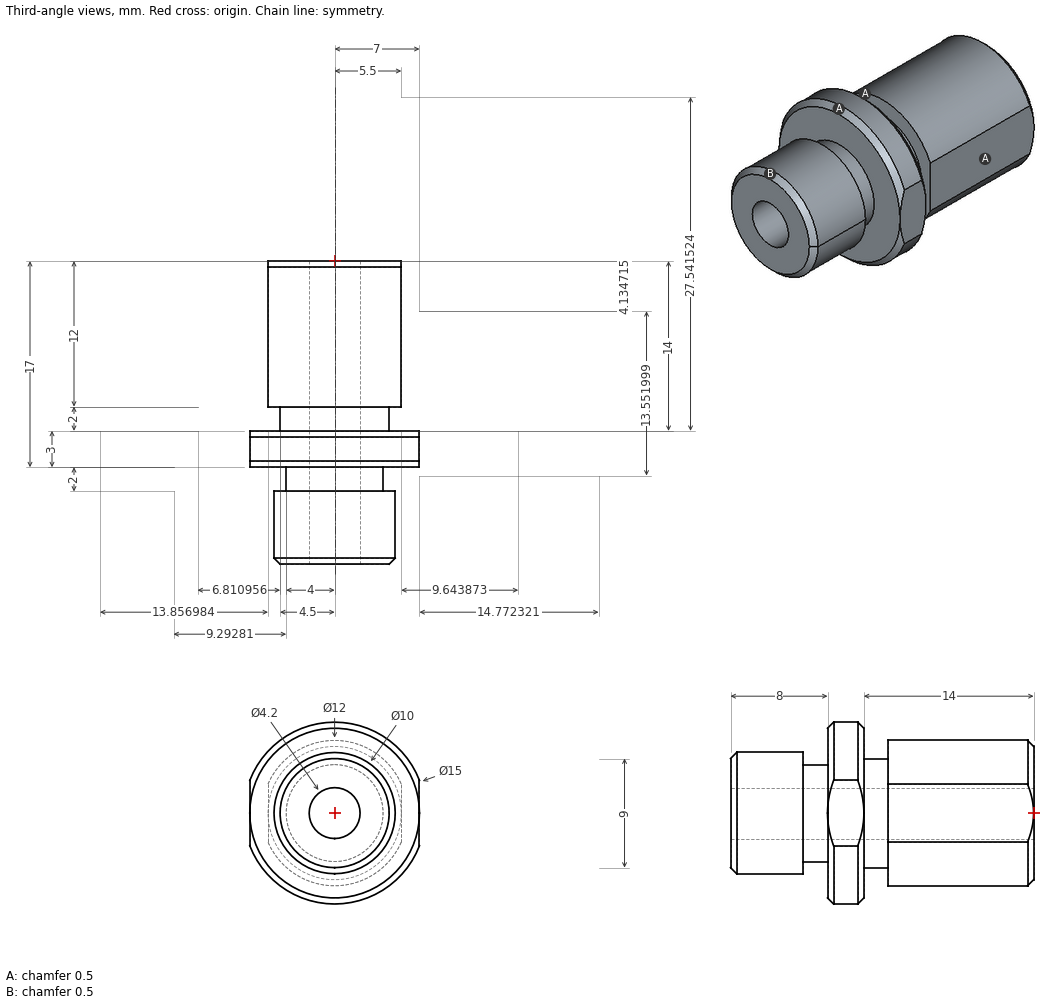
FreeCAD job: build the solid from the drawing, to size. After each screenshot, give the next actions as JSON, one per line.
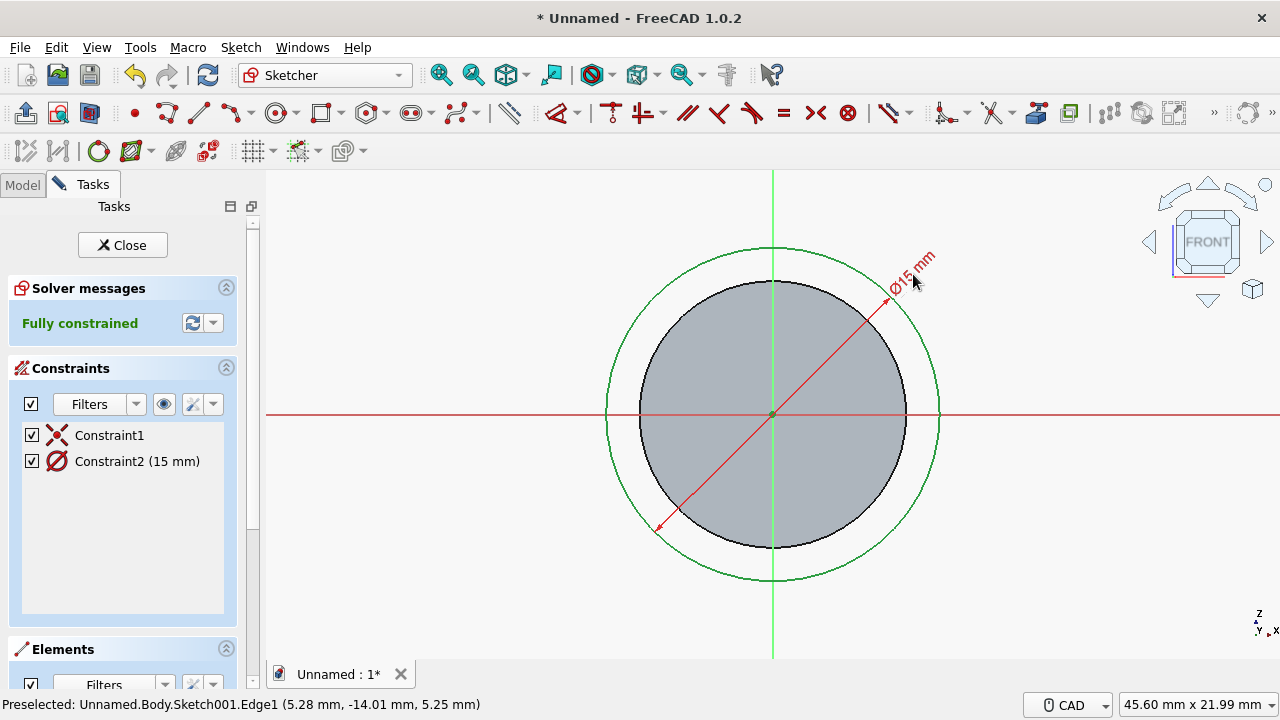
{"action": "left_click", "coordinate": [123, 245]}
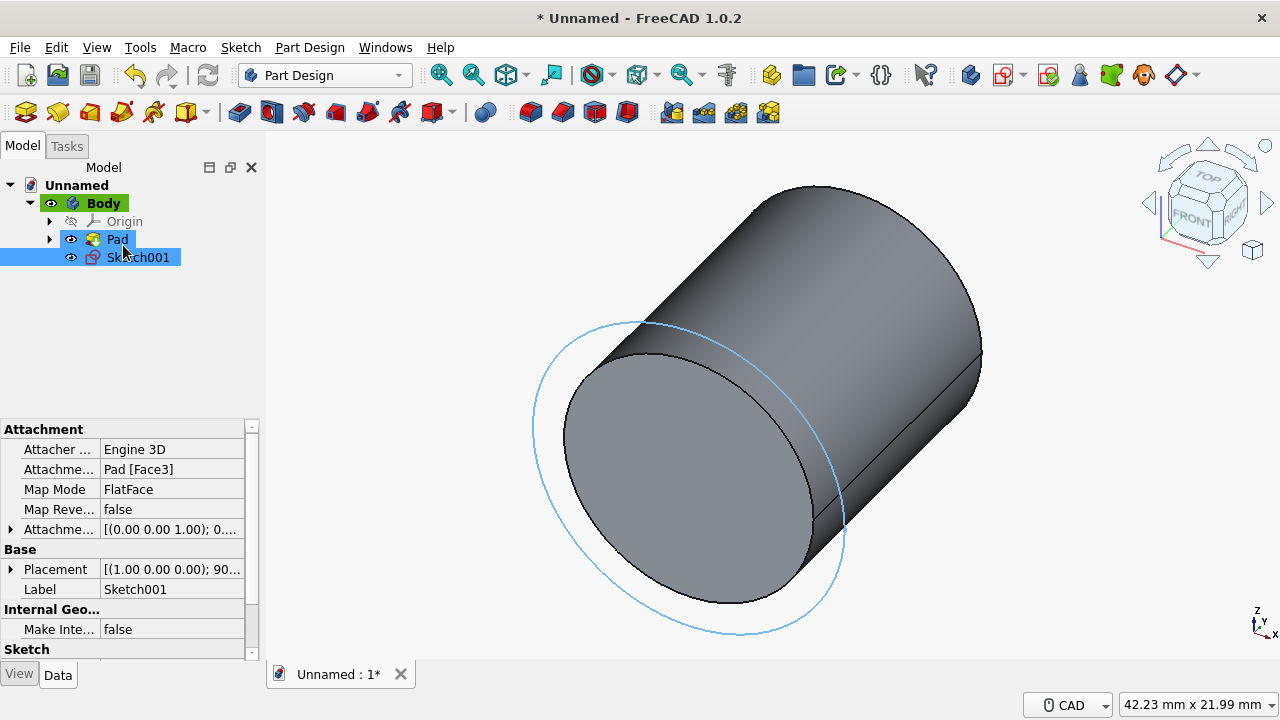
{"action": "left_click", "coordinate": [26, 112]}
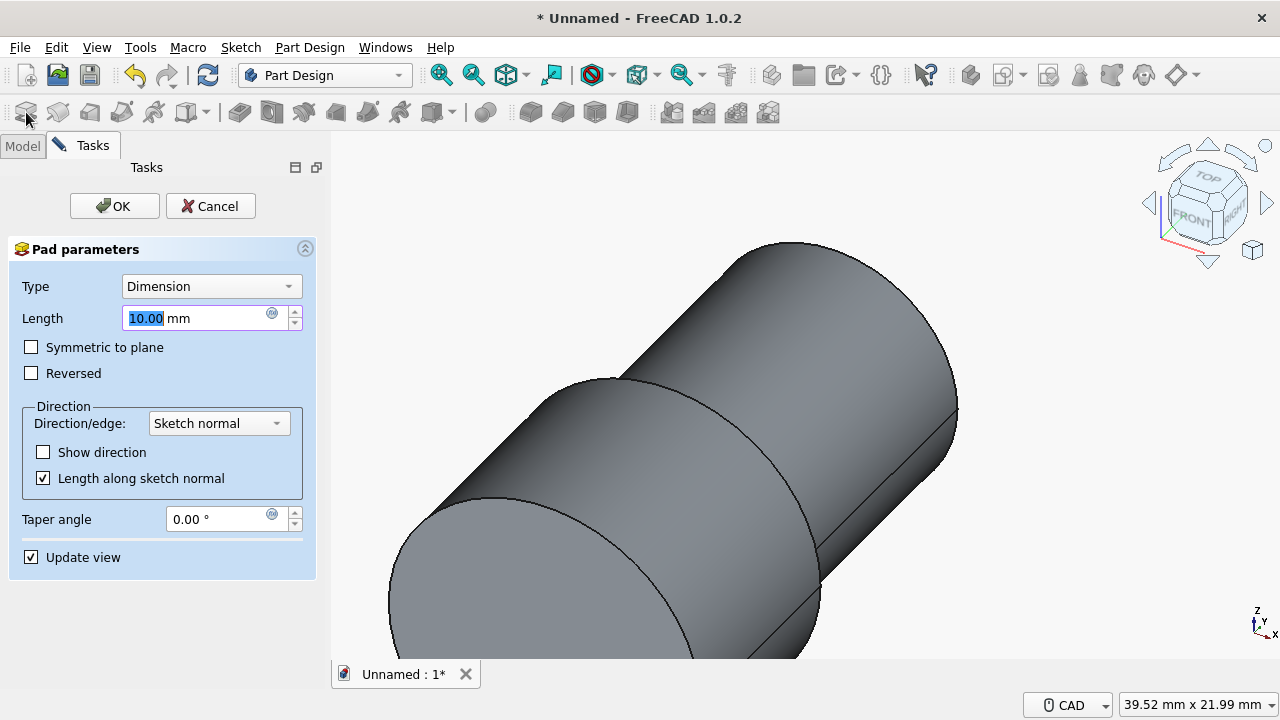
{"action": "type", "text": "3"}
{"action": "key", "text": "Tab"}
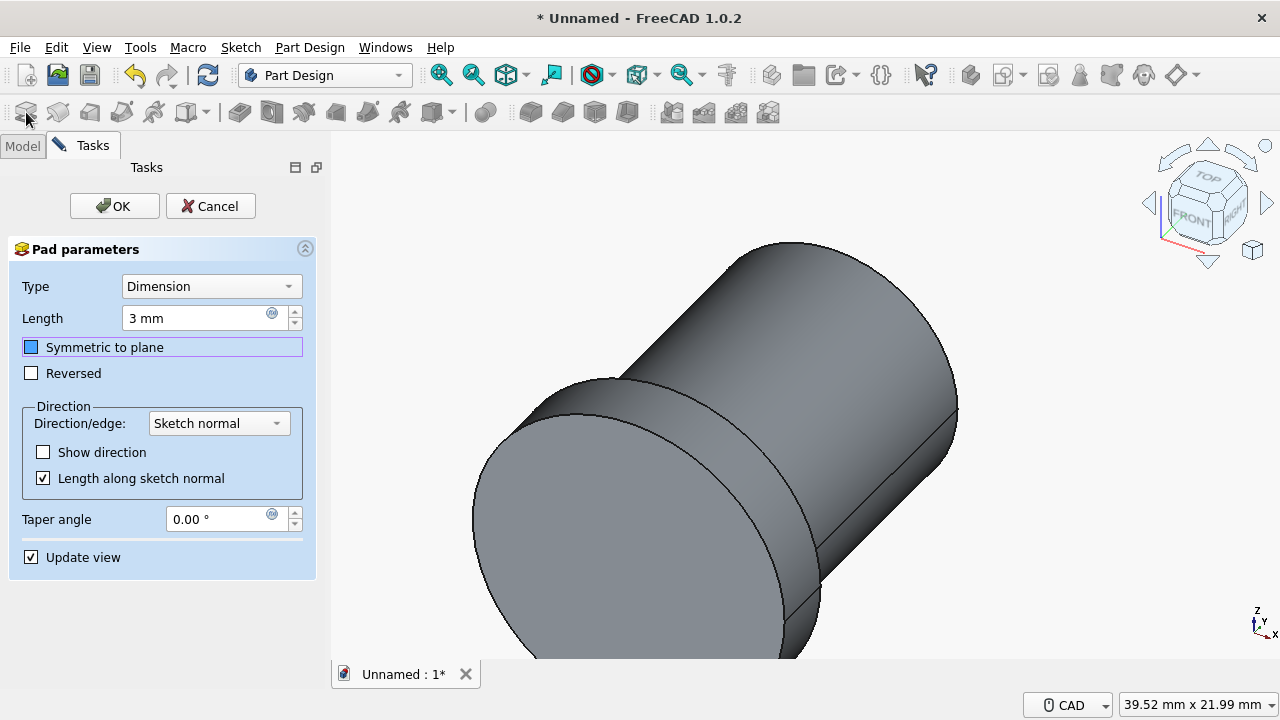
{"action": "left_click", "coordinate": [115, 206]}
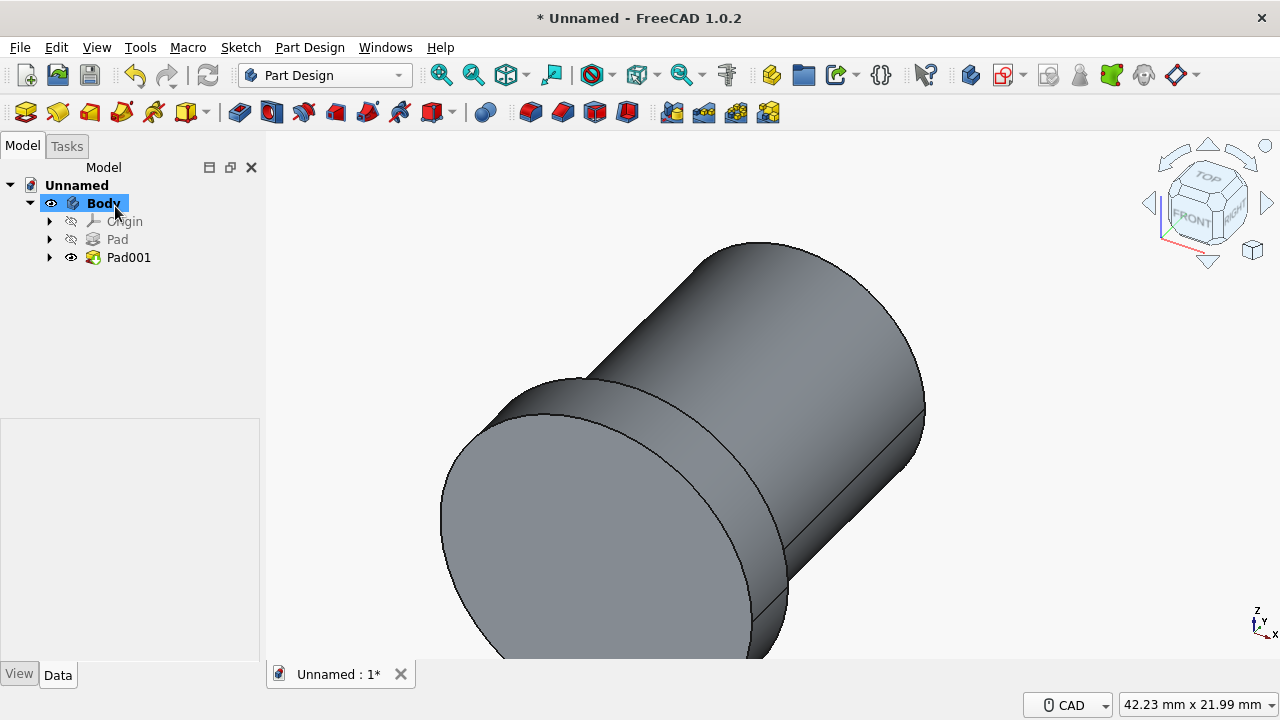
{"action": "key", "text": "v f"}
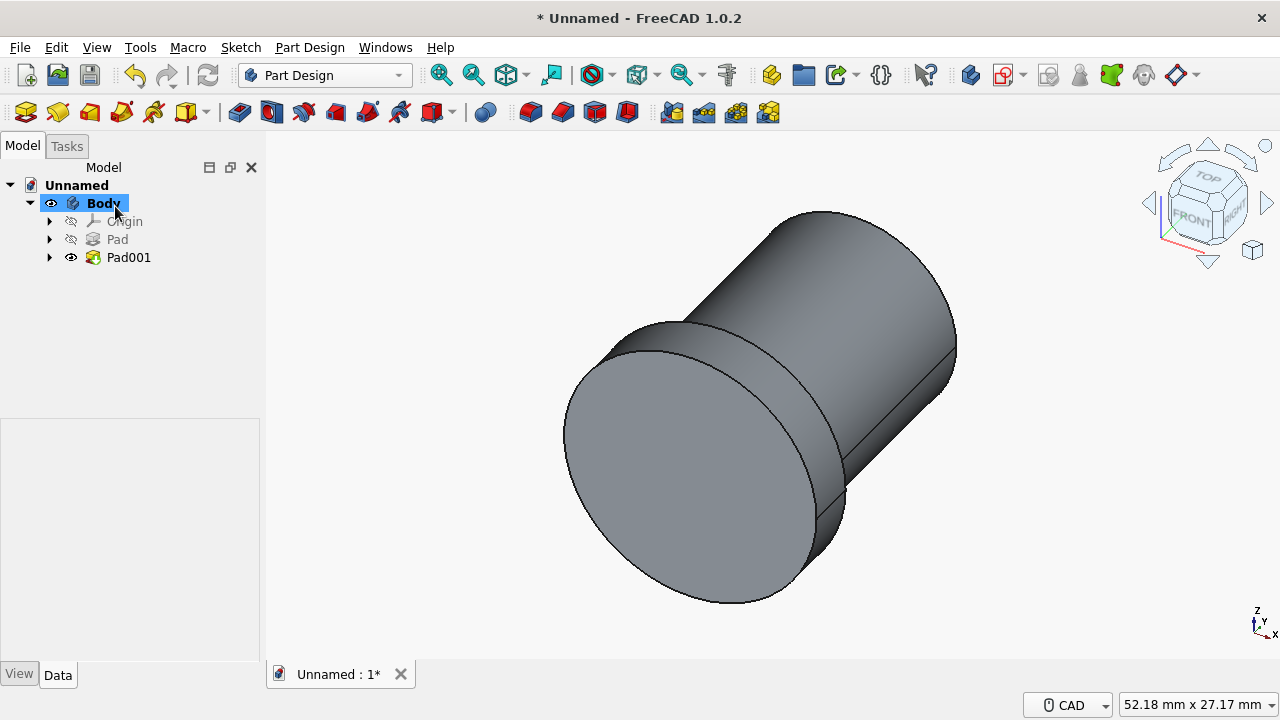
{"action": "left_click", "coordinate": [690, 476]}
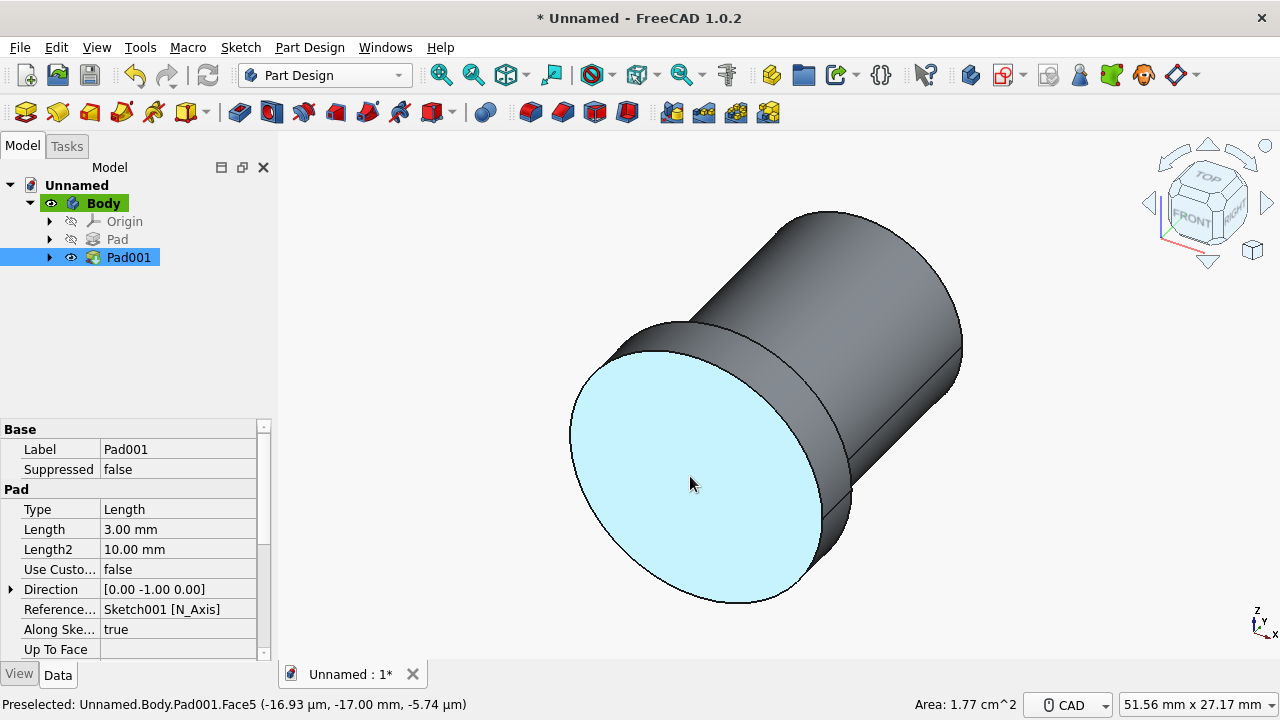
{"action": "left_click", "coordinate": [1004, 76]}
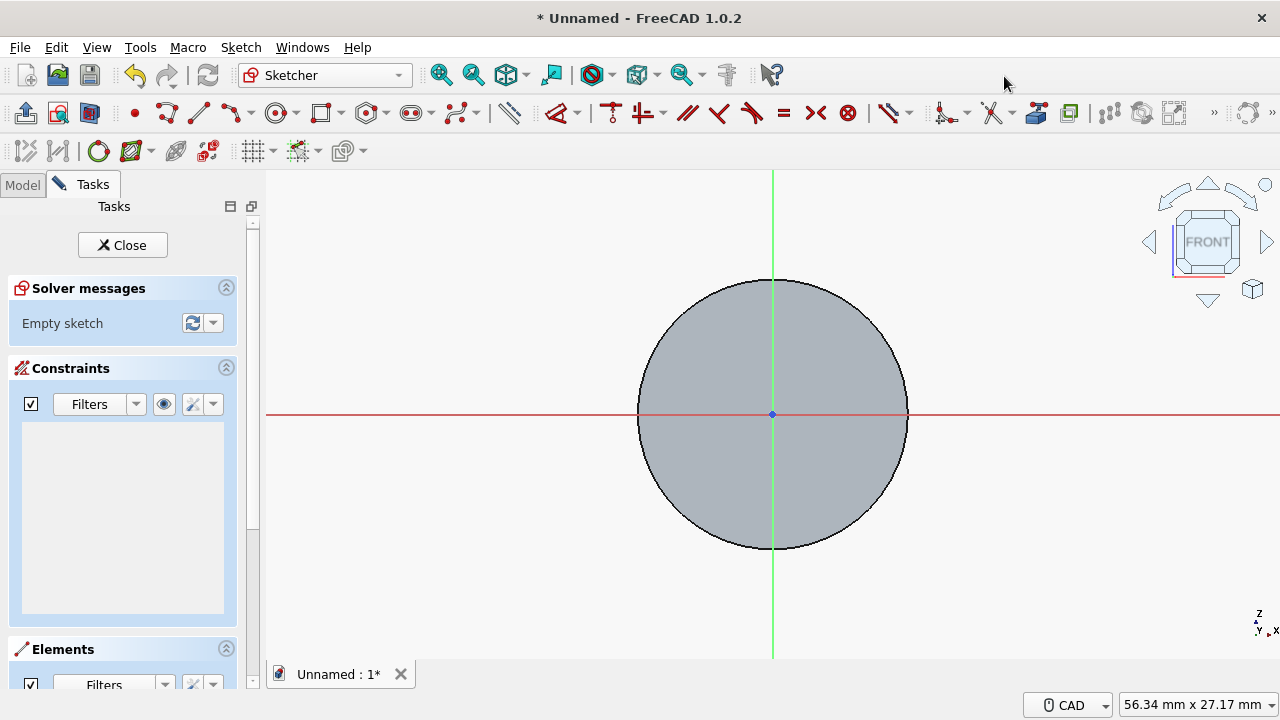
{"action": "scroll", "coordinate": [856, 414], "scroll_direction": "up", "scroll_amount": 3}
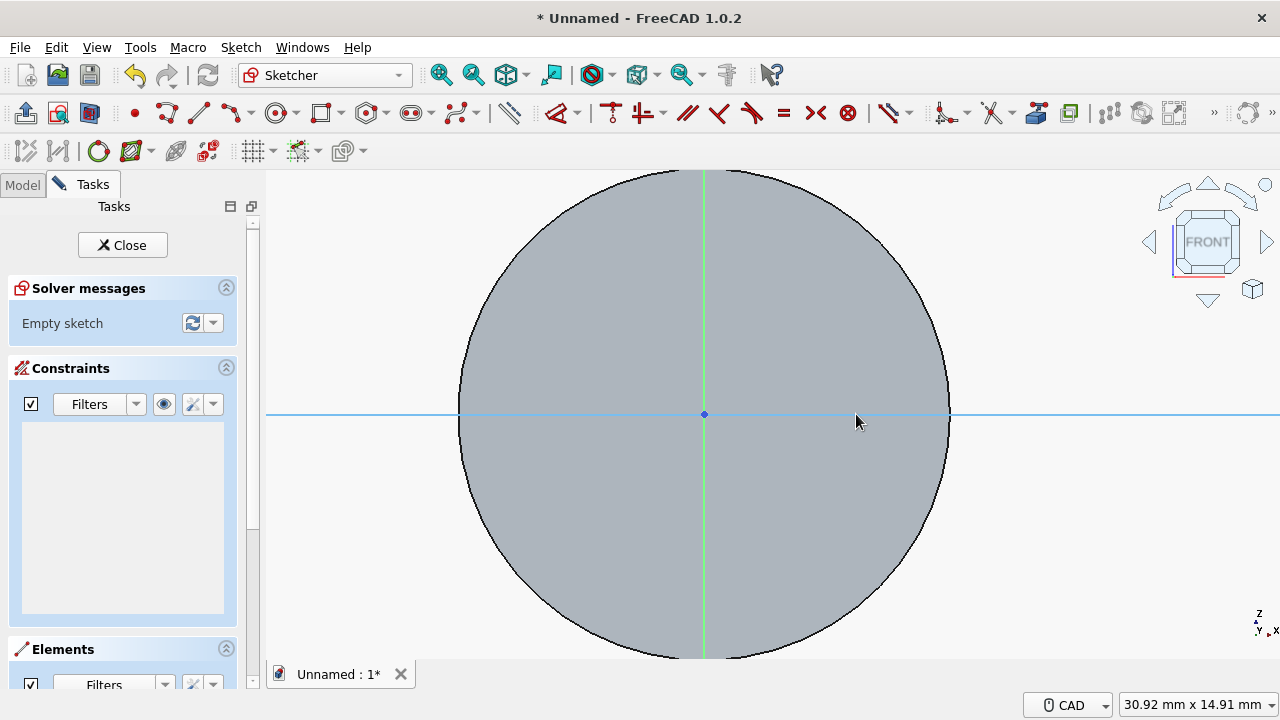
{"action": "key", "text": "g c"}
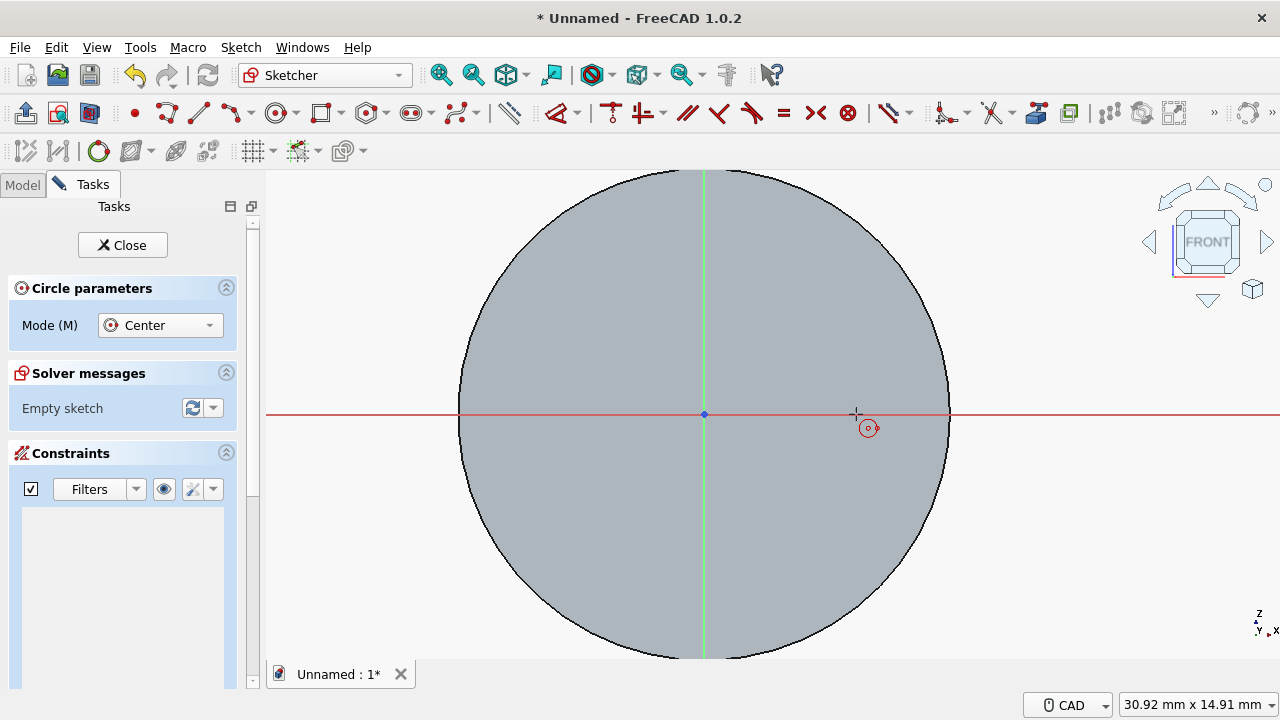
{"action": "left_click", "coordinate": [704, 414]}
{"action": "left_click", "coordinate": [820, 299]}
{"action": "key", "text": "Escape"}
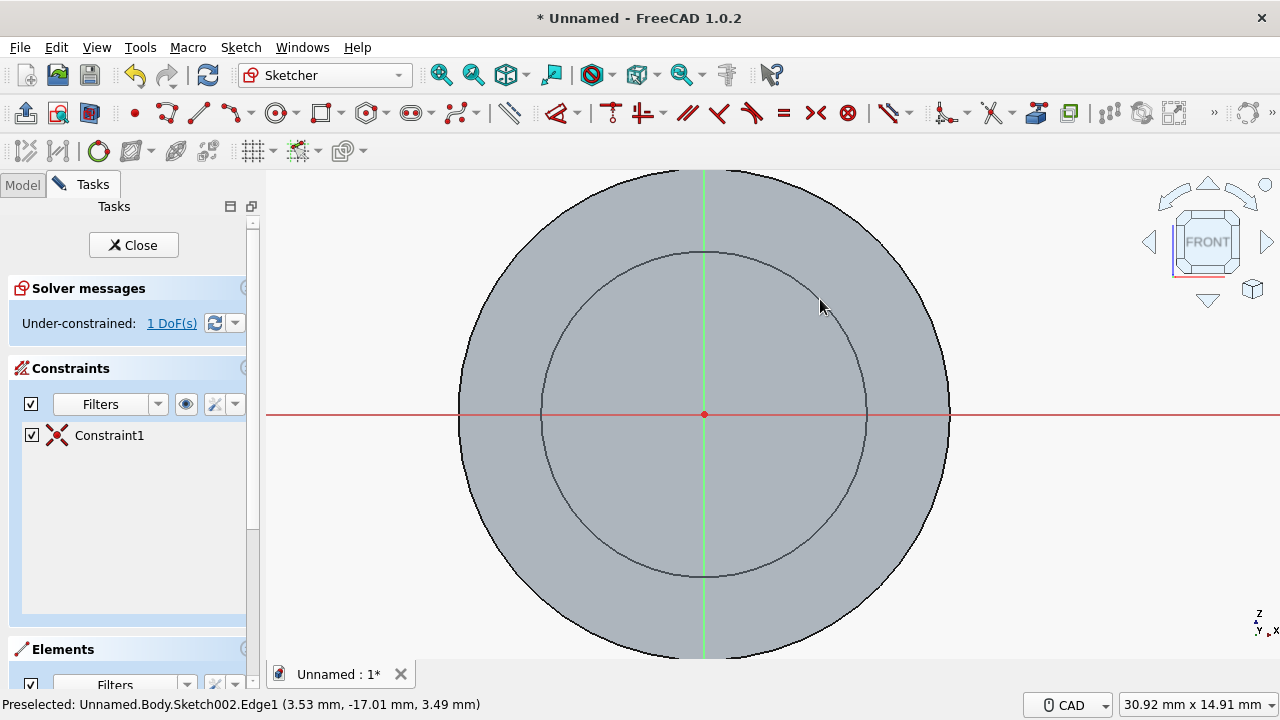
{"action": "key", "text": "d"}